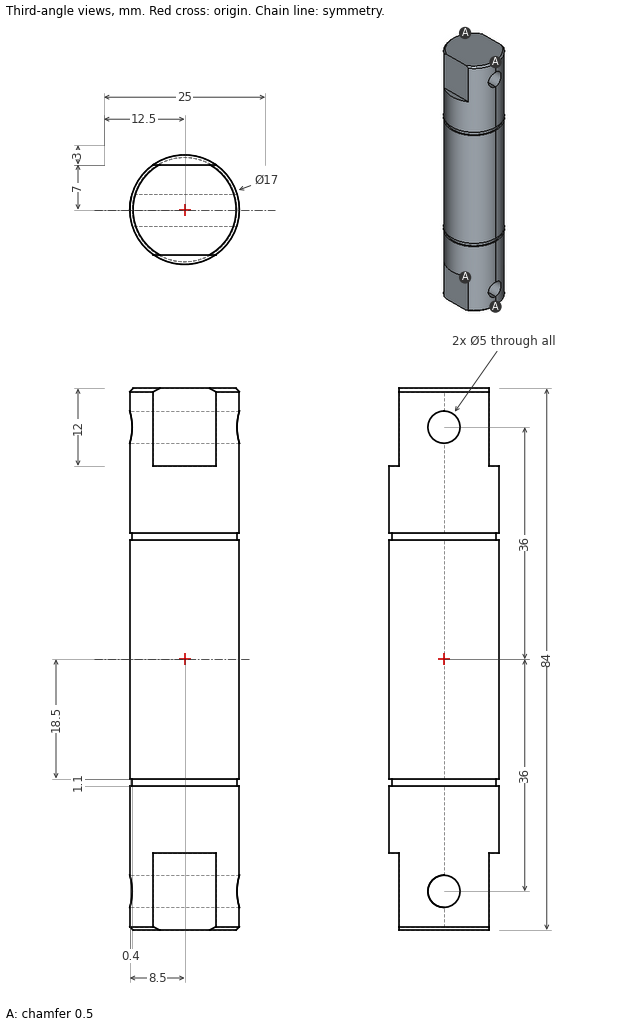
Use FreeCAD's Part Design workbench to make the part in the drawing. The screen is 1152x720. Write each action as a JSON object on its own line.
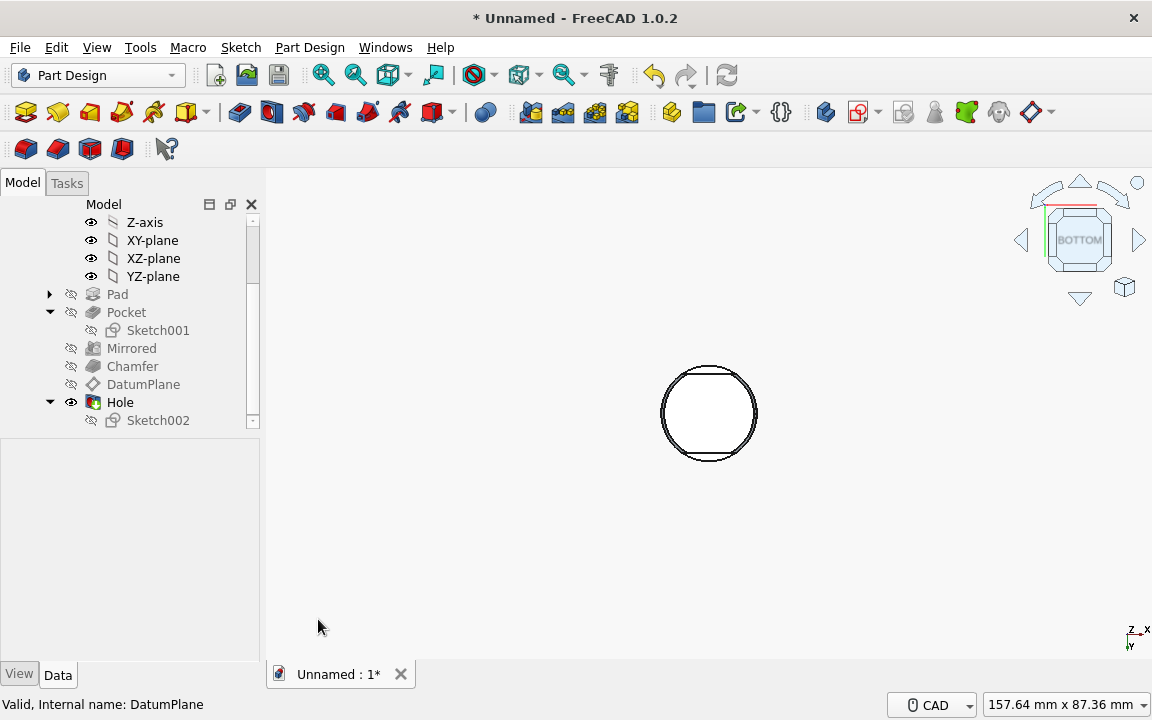
{"action": "left_click", "coordinate": [858, 112]}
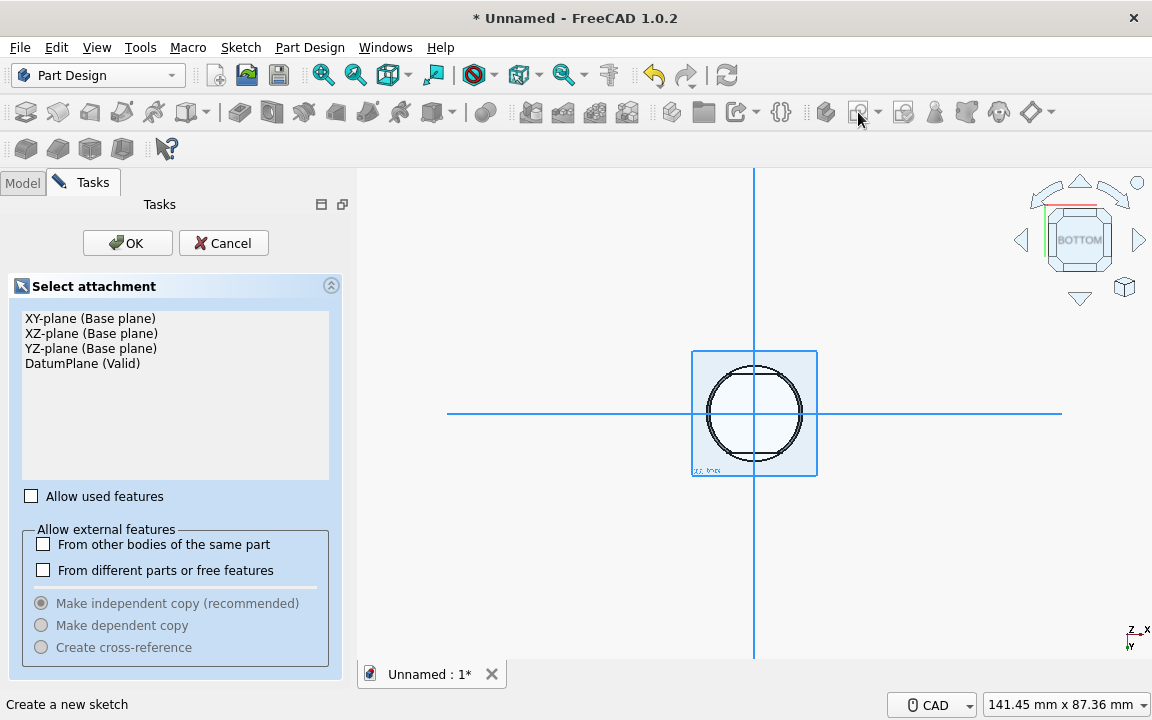
{"action": "left_click", "coordinate": [82, 334]}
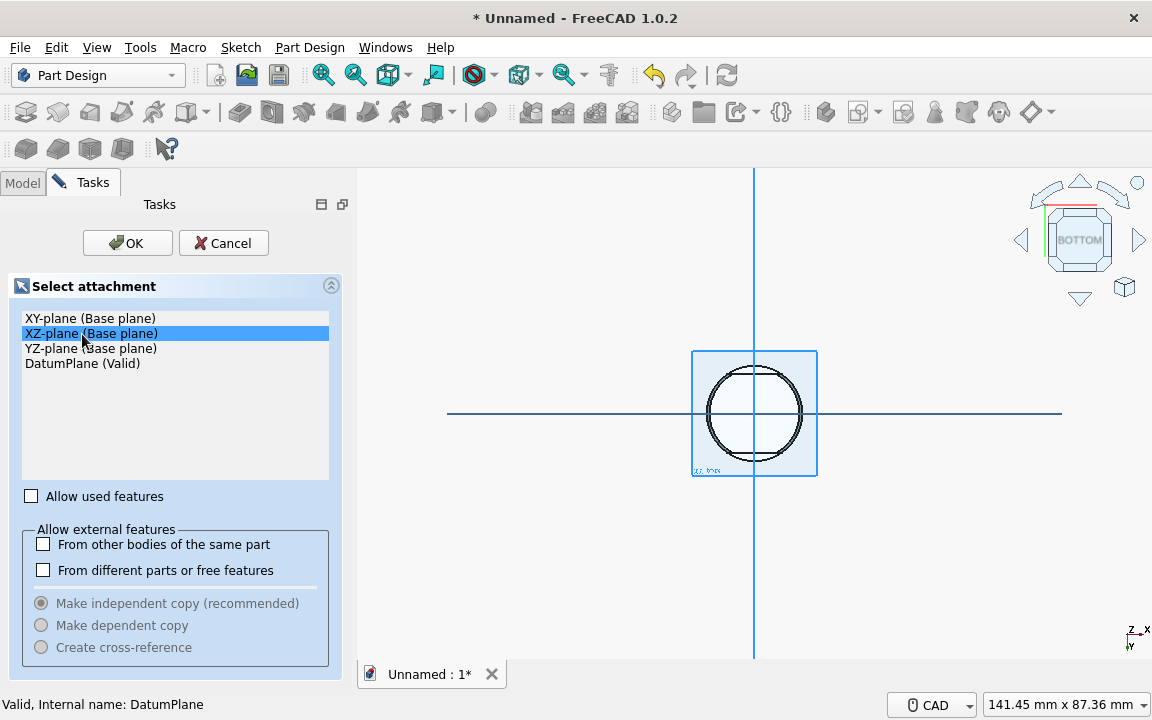
{"action": "left_click", "coordinate": [128, 243]}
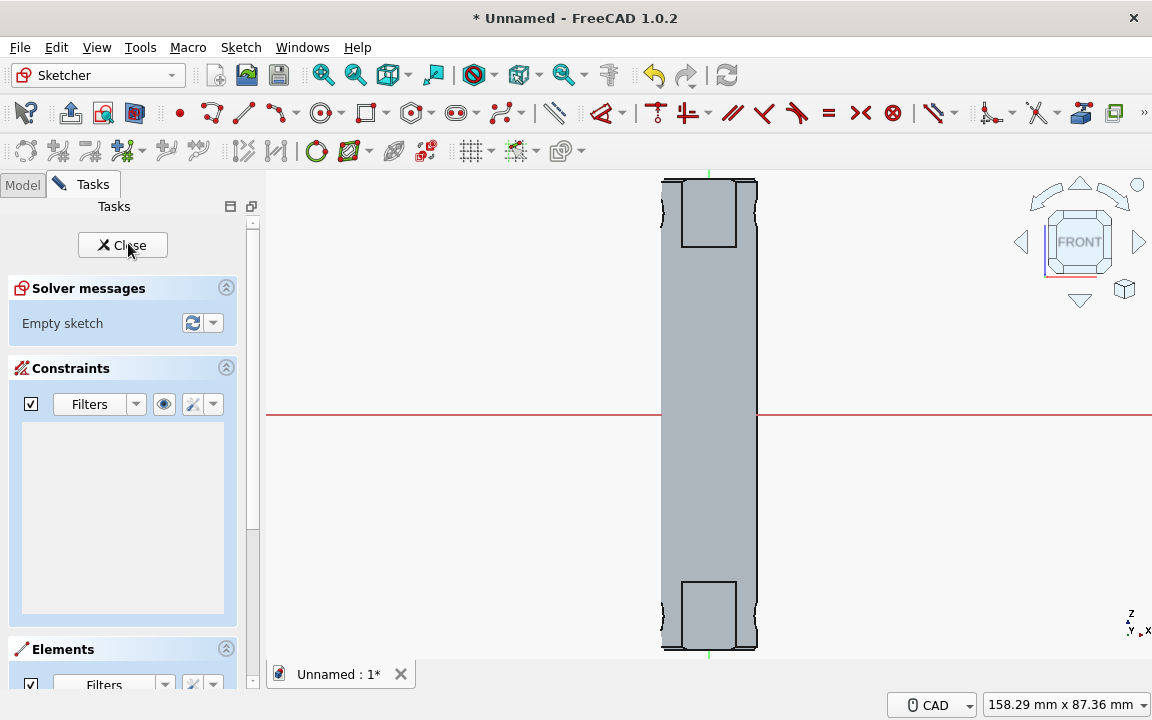
{"action": "left_click", "coordinate": [136, 114]}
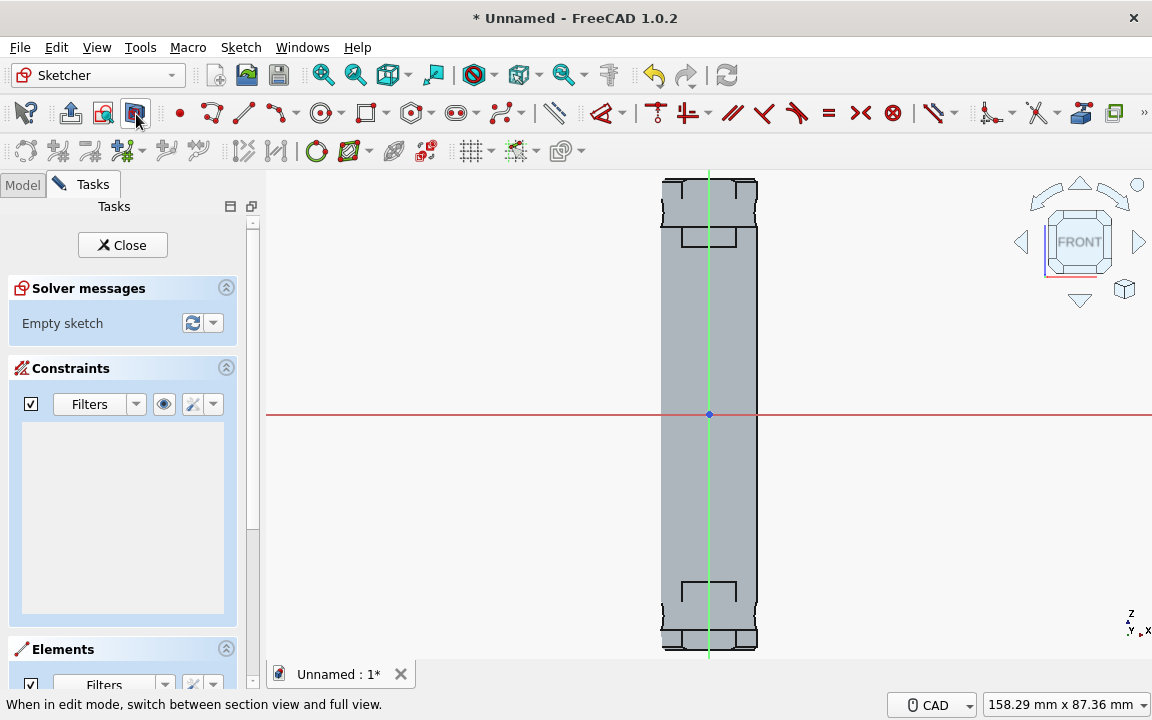
{"action": "scroll", "coordinate": [776, 415], "scroll_direction": "up", "scroll_amount": 2}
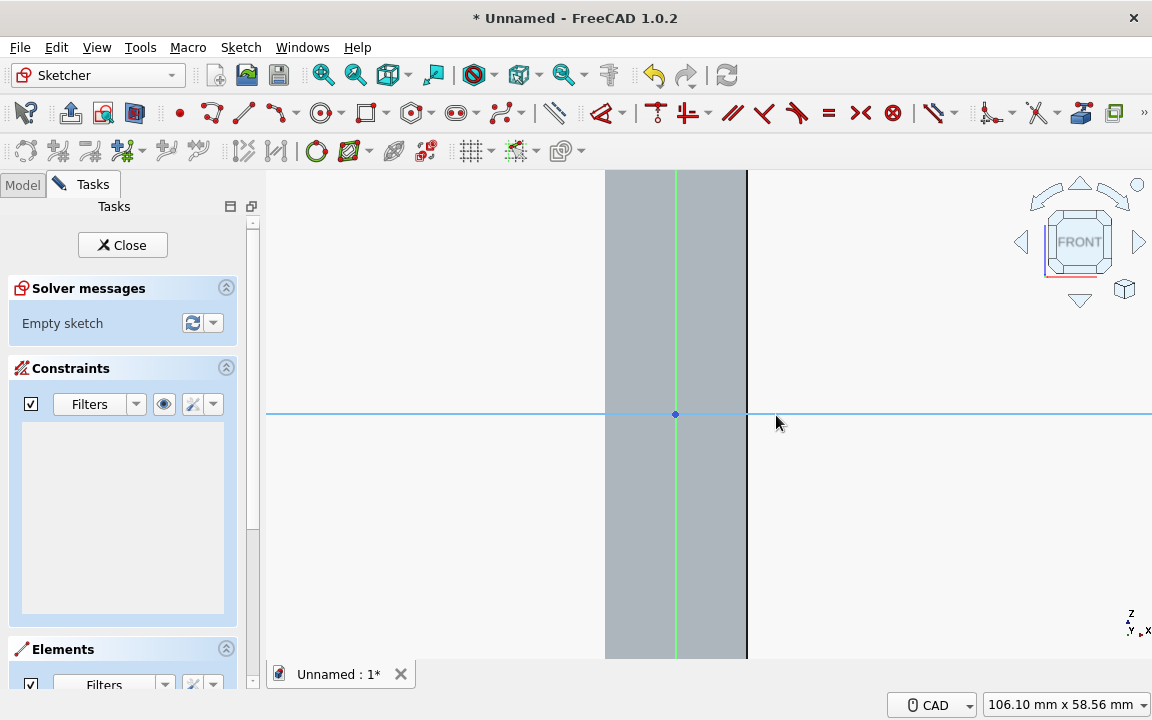
{"action": "left_click", "coordinate": [366, 114]}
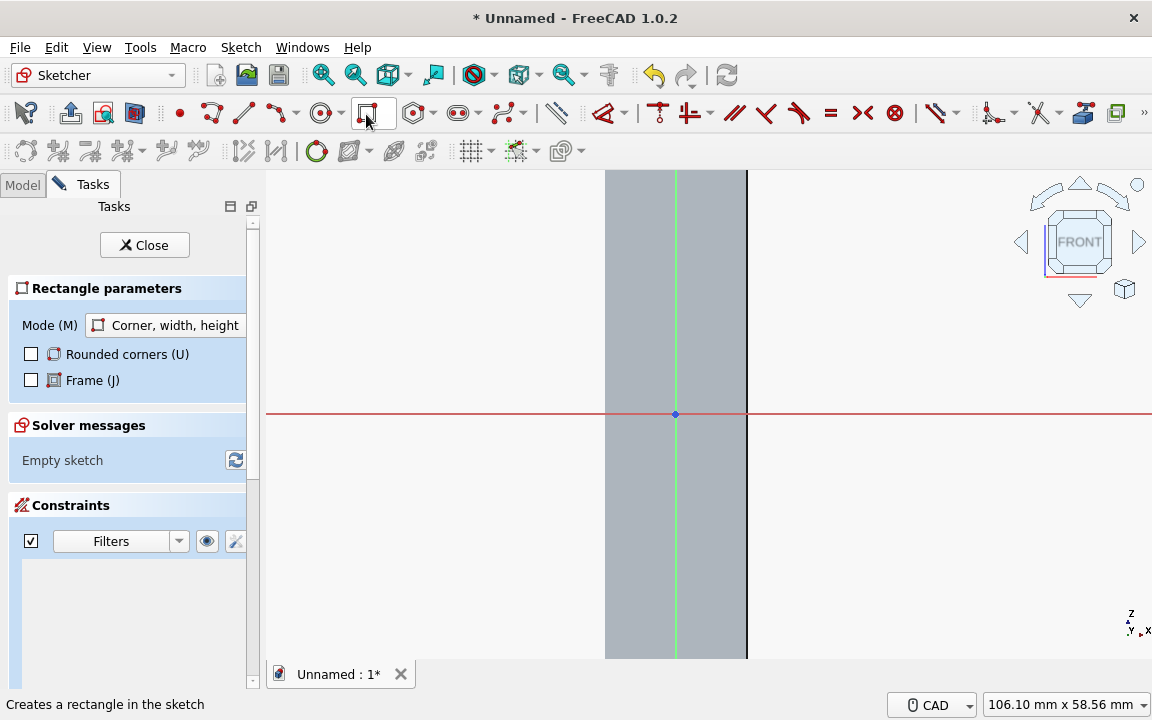
{"action": "scroll", "coordinate": [605, 568], "scroll_direction": "up", "scroll_amount": 8}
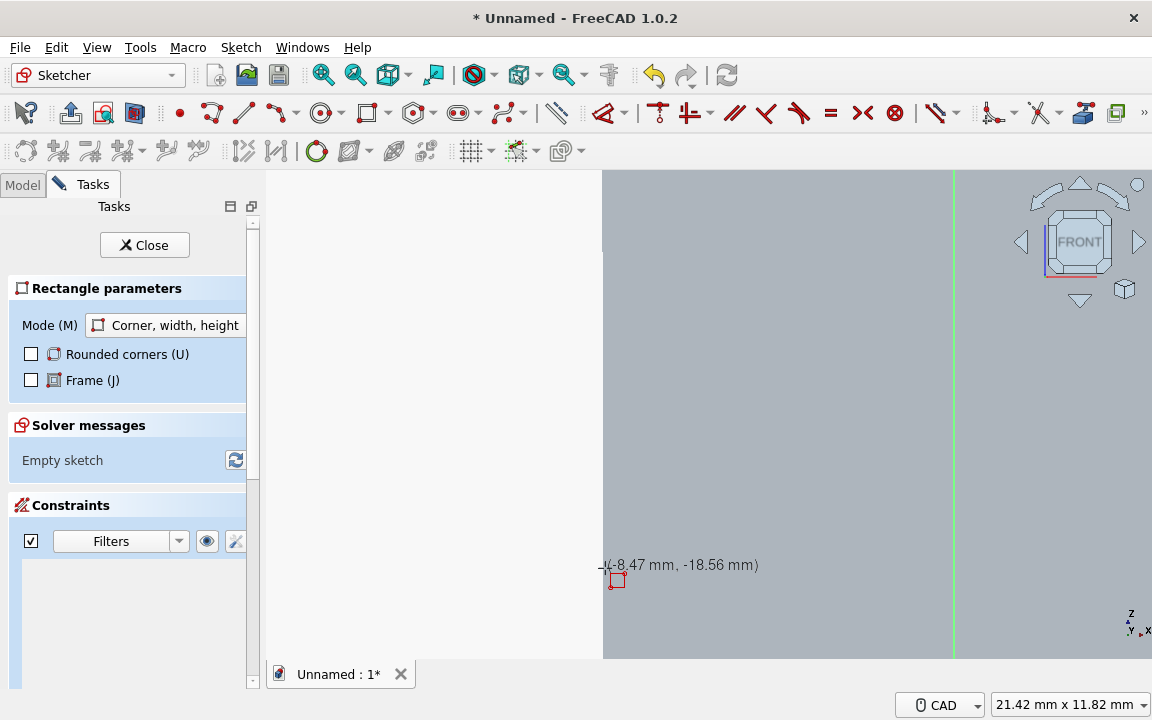
{"action": "scroll", "coordinate": [606, 569], "scroll_direction": "down", "scroll_amount": 8}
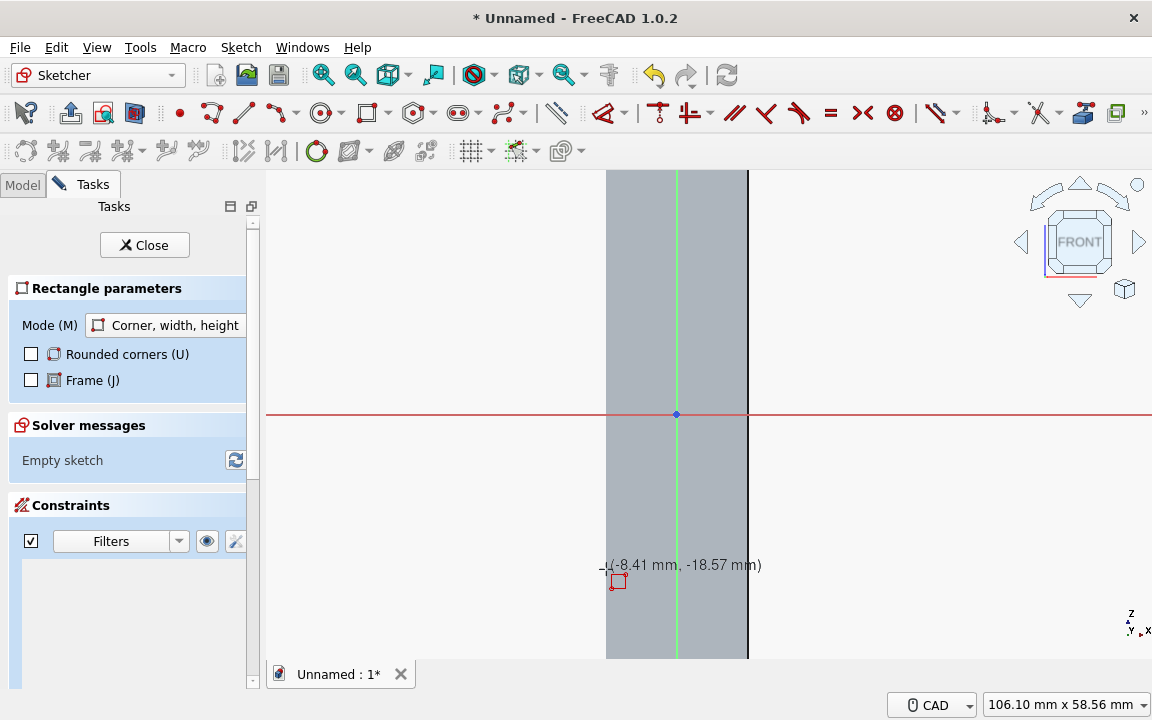
{"action": "left_click", "coordinate": [606, 569]}
{"action": "left_click", "coordinate": [609, 578]}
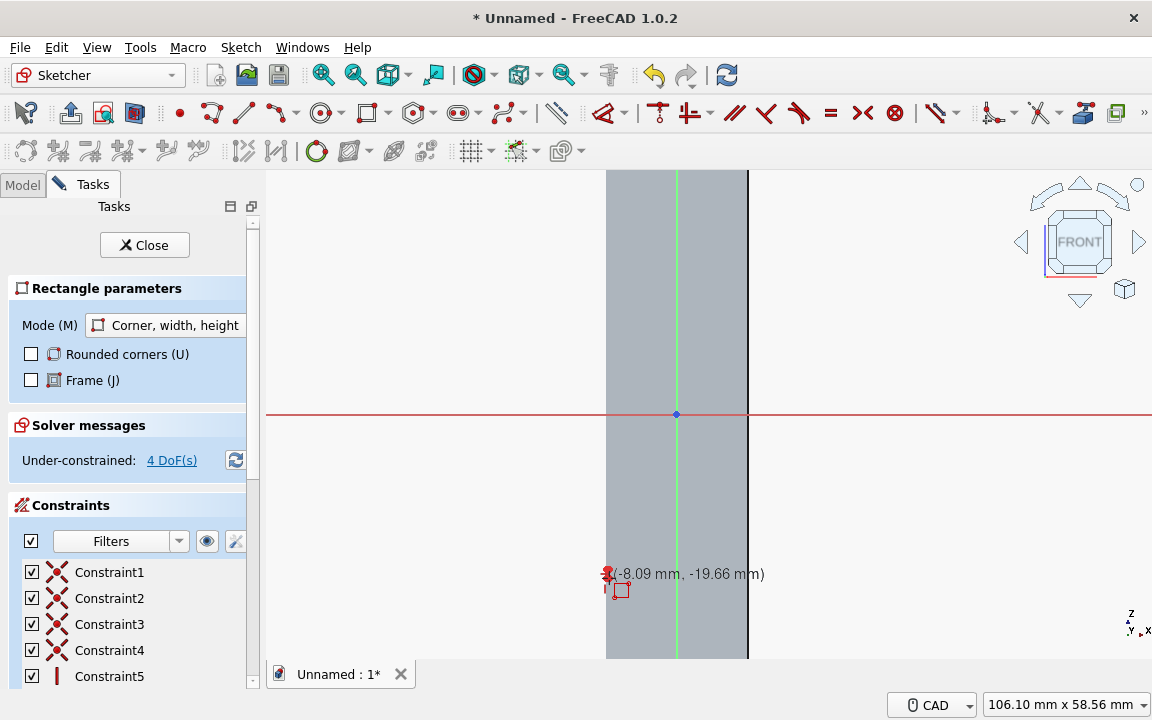
{"action": "scroll", "coordinate": [606, 251], "scroll_direction": "up", "scroll_amount": 8}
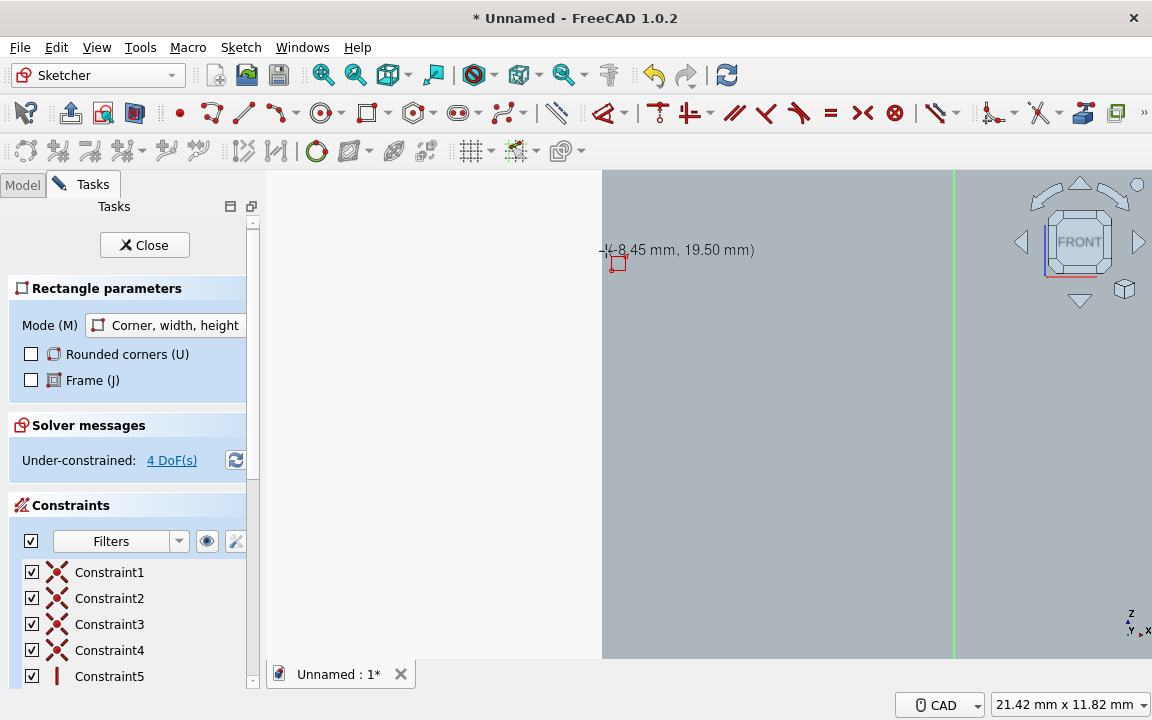
{"action": "scroll", "coordinate": [606, 251], "scroll_direction": "down", "scroll_amount": 8}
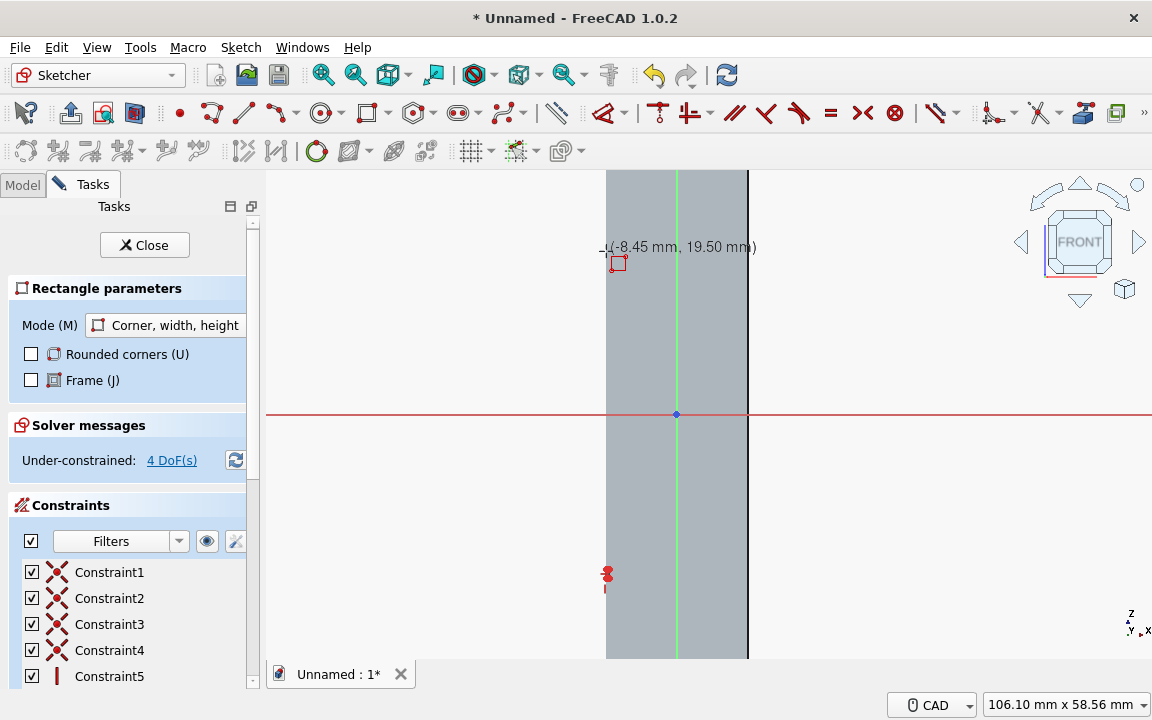
{"action": "left_click", "coordinate": [606, 251]}
{"action": "left_click", "coordinate": [609, 260]}
{"action": "key", "text": "Escape"}